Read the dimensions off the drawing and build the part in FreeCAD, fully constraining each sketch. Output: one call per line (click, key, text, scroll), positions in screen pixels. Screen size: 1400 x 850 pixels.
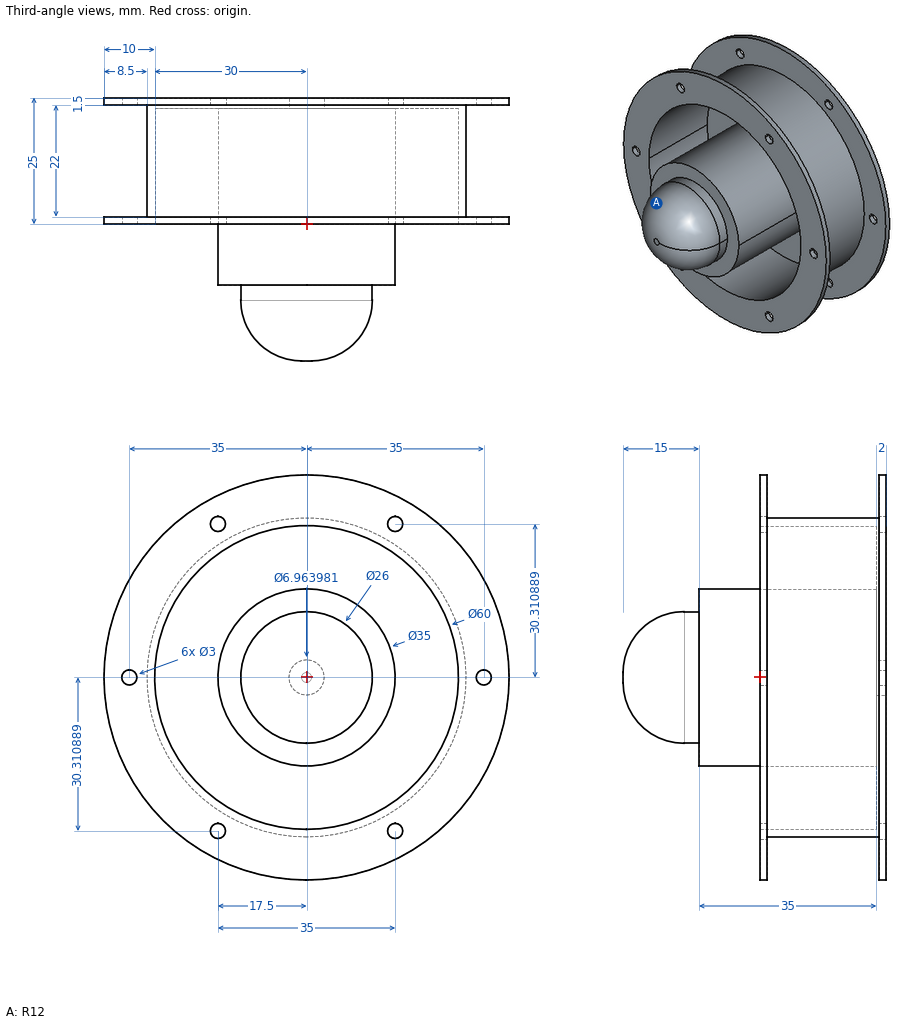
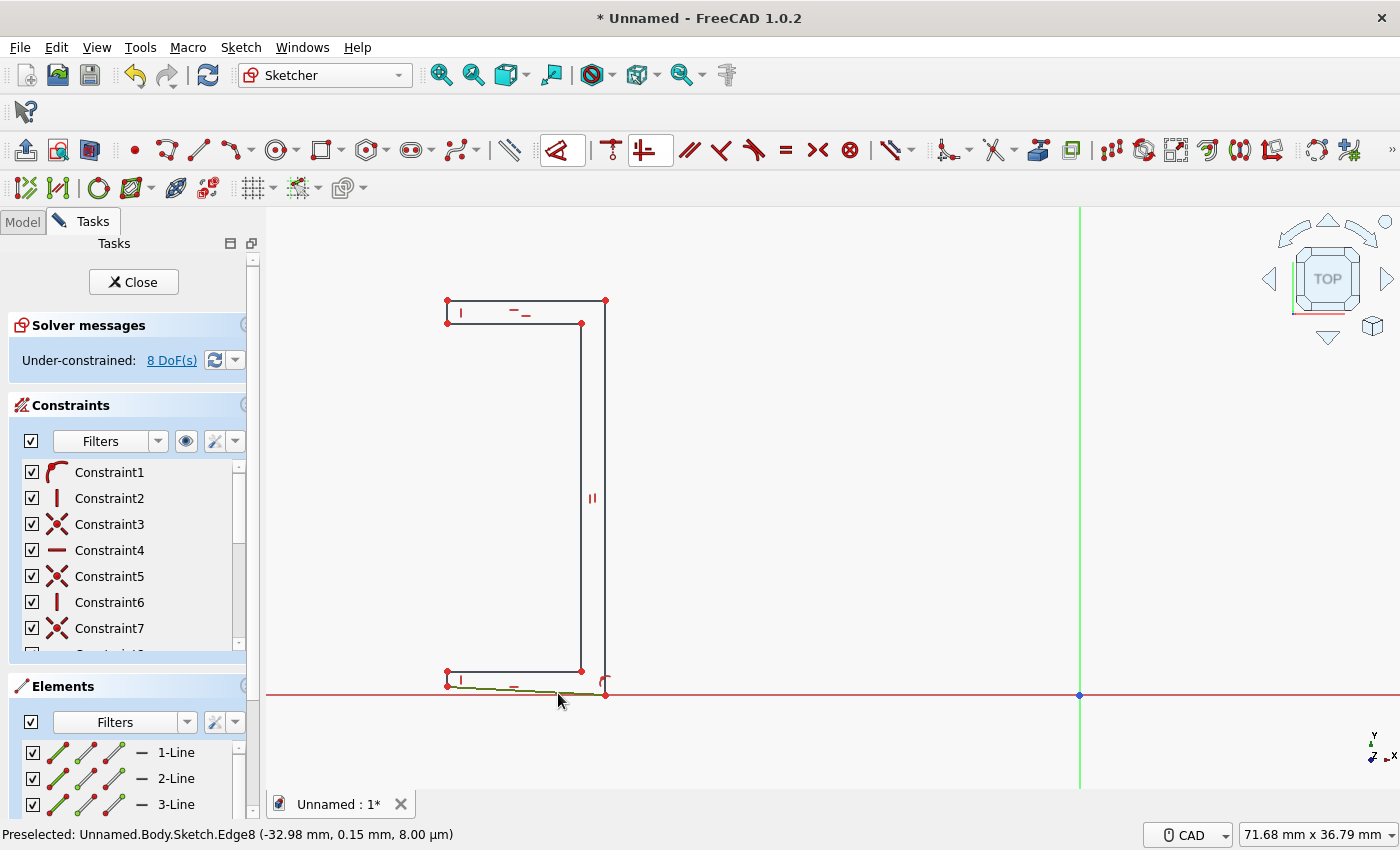
key(h)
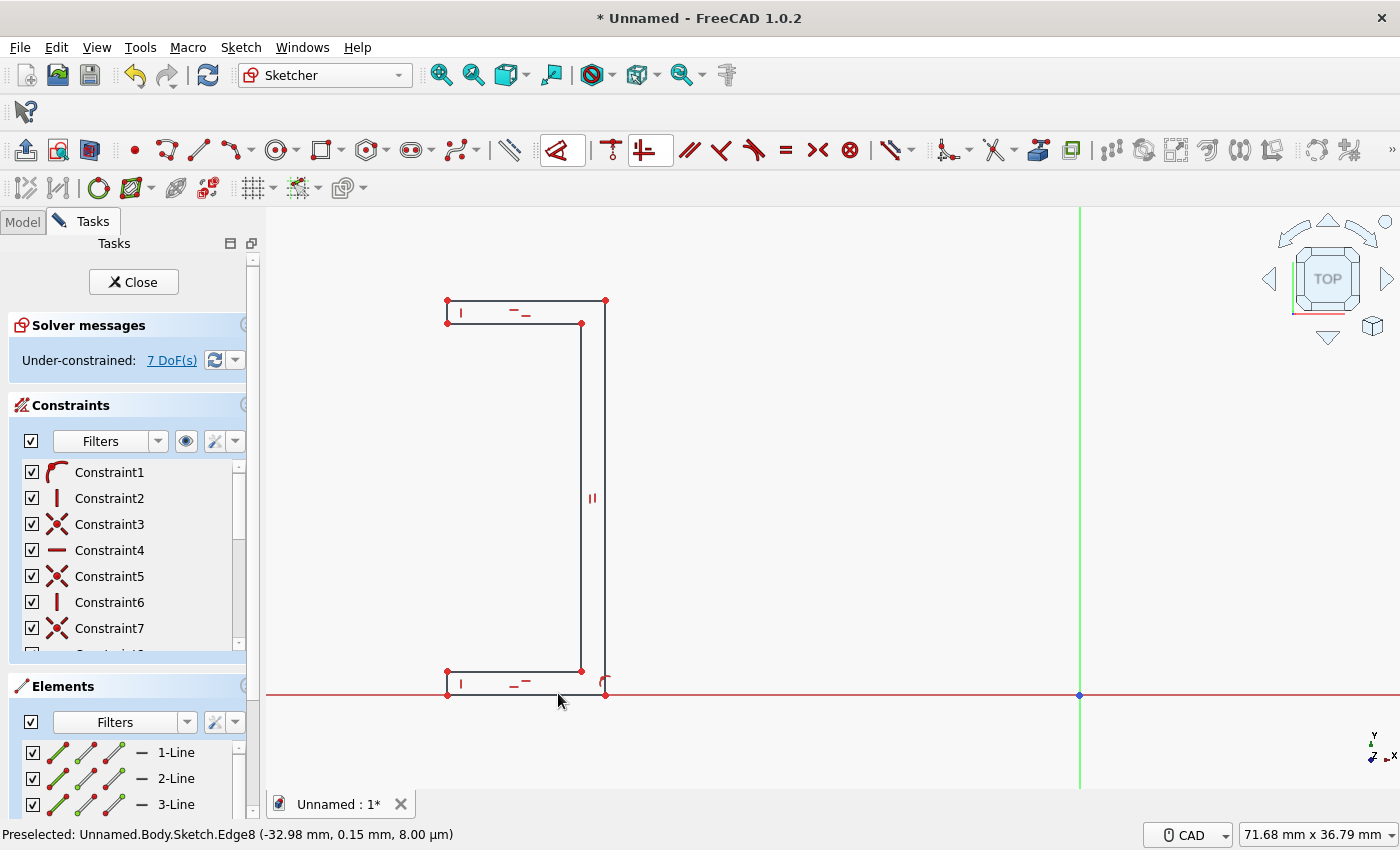
click(556, 150)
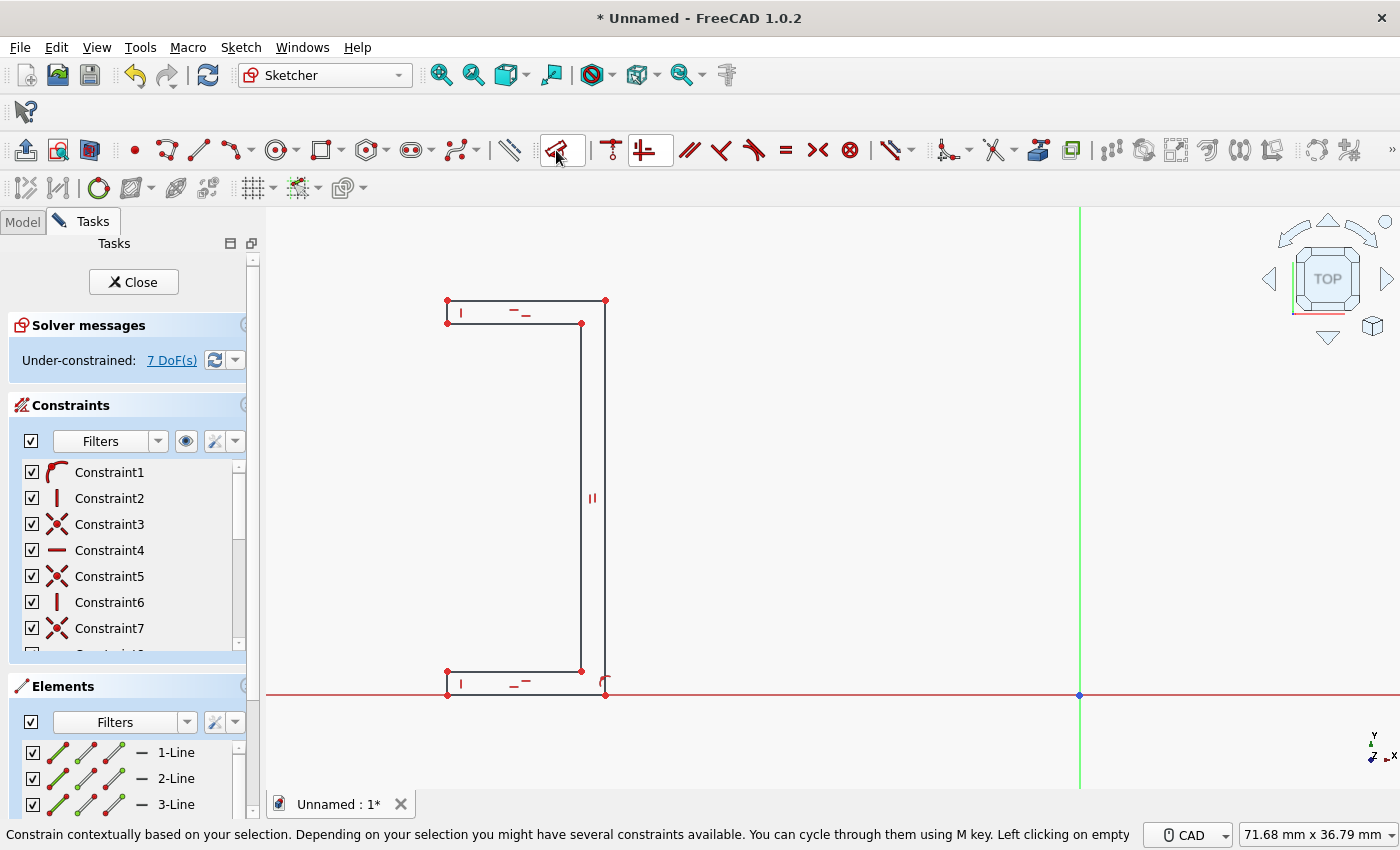
click(605, 577)
click(639, 498)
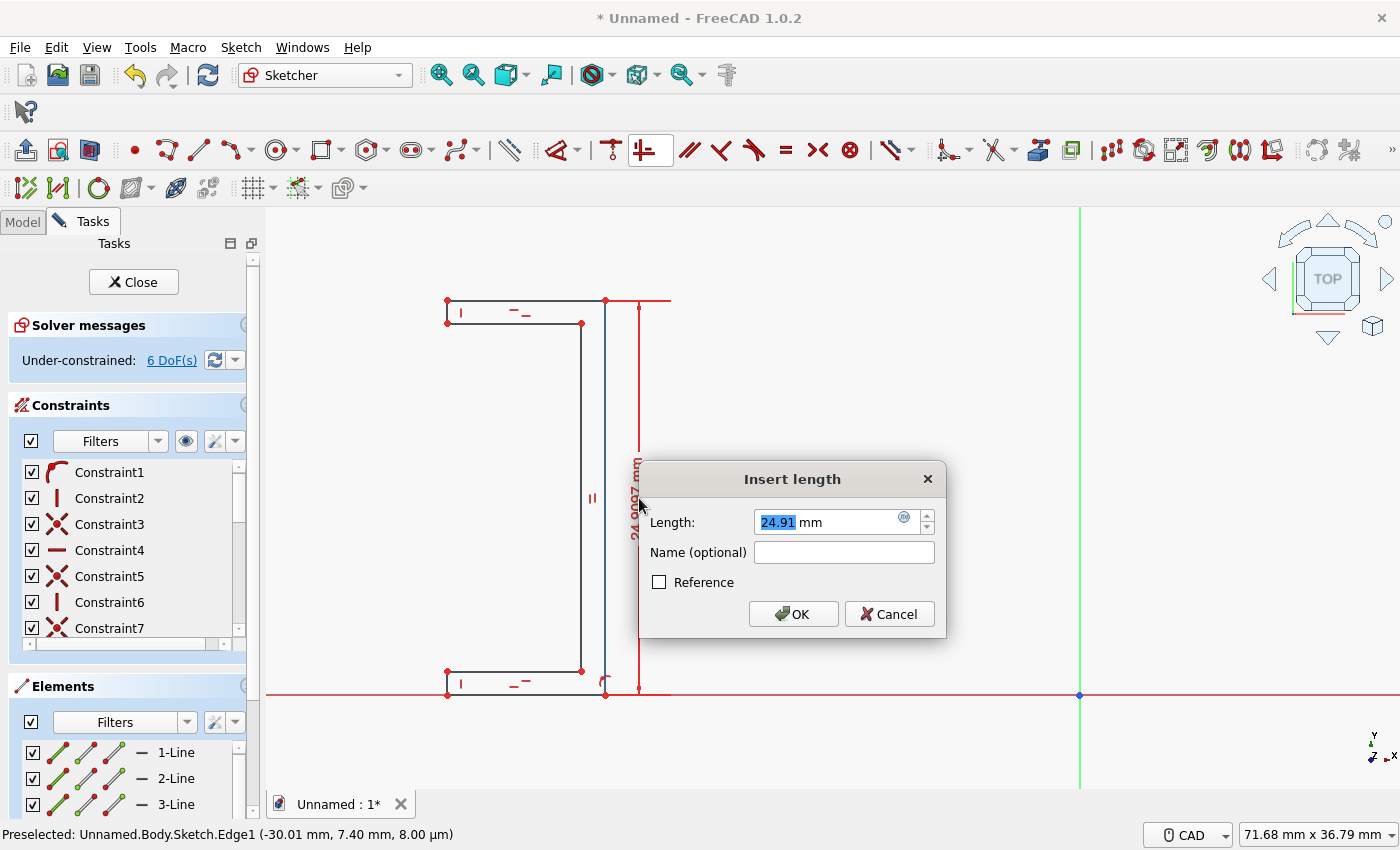
text(25)
key(Return)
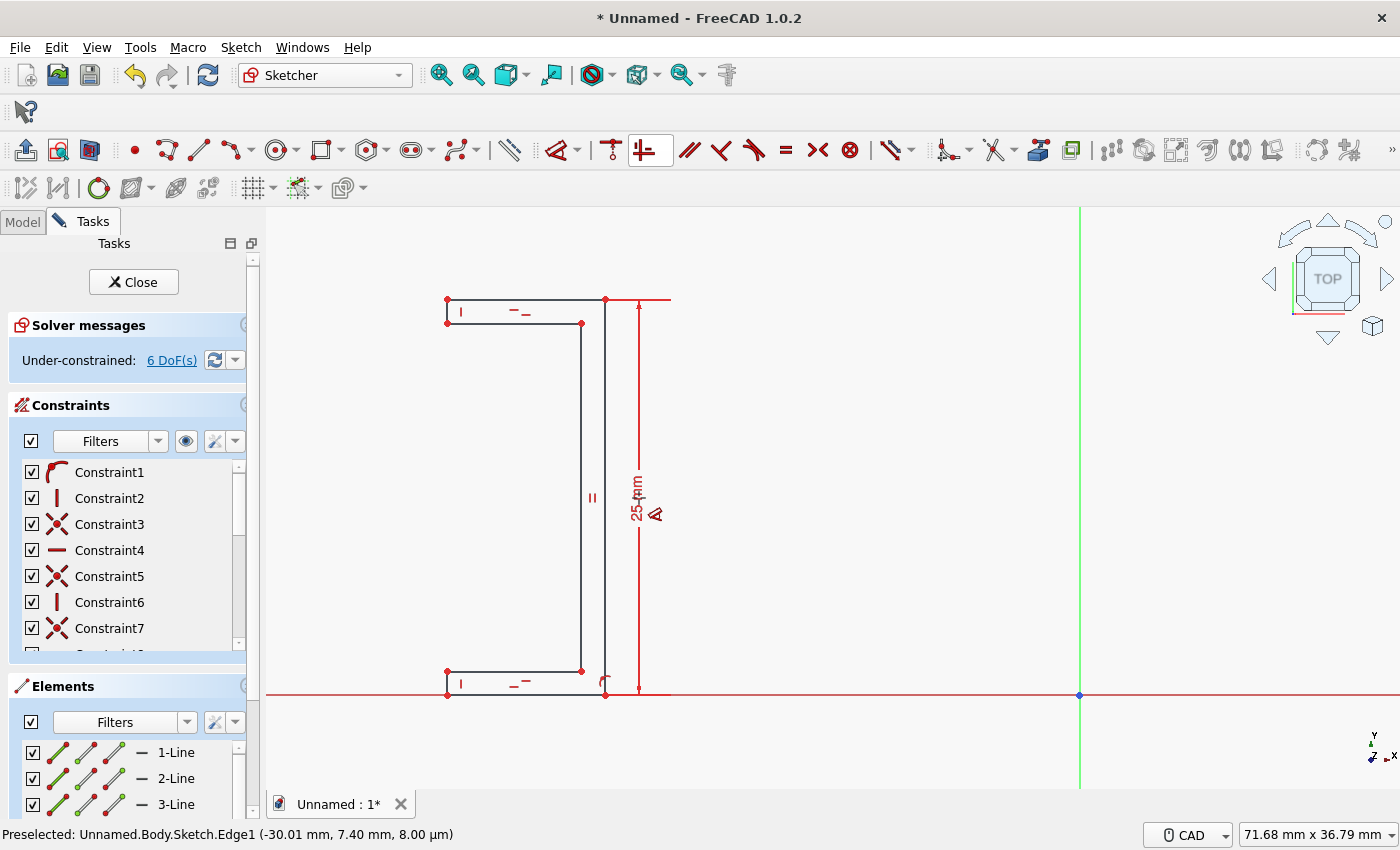
click(558, 300)
click(526, 266)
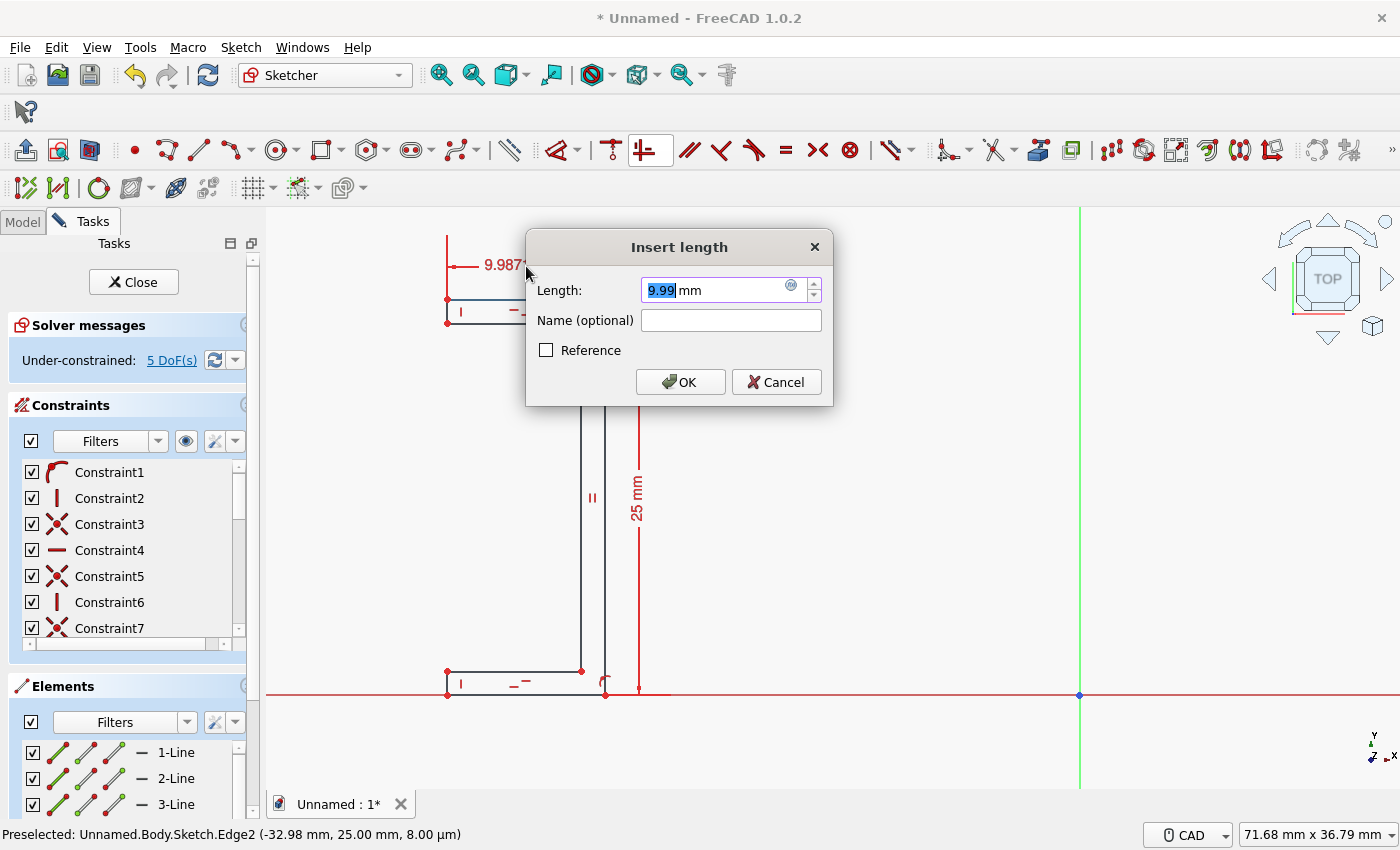
text(10)
key(Return)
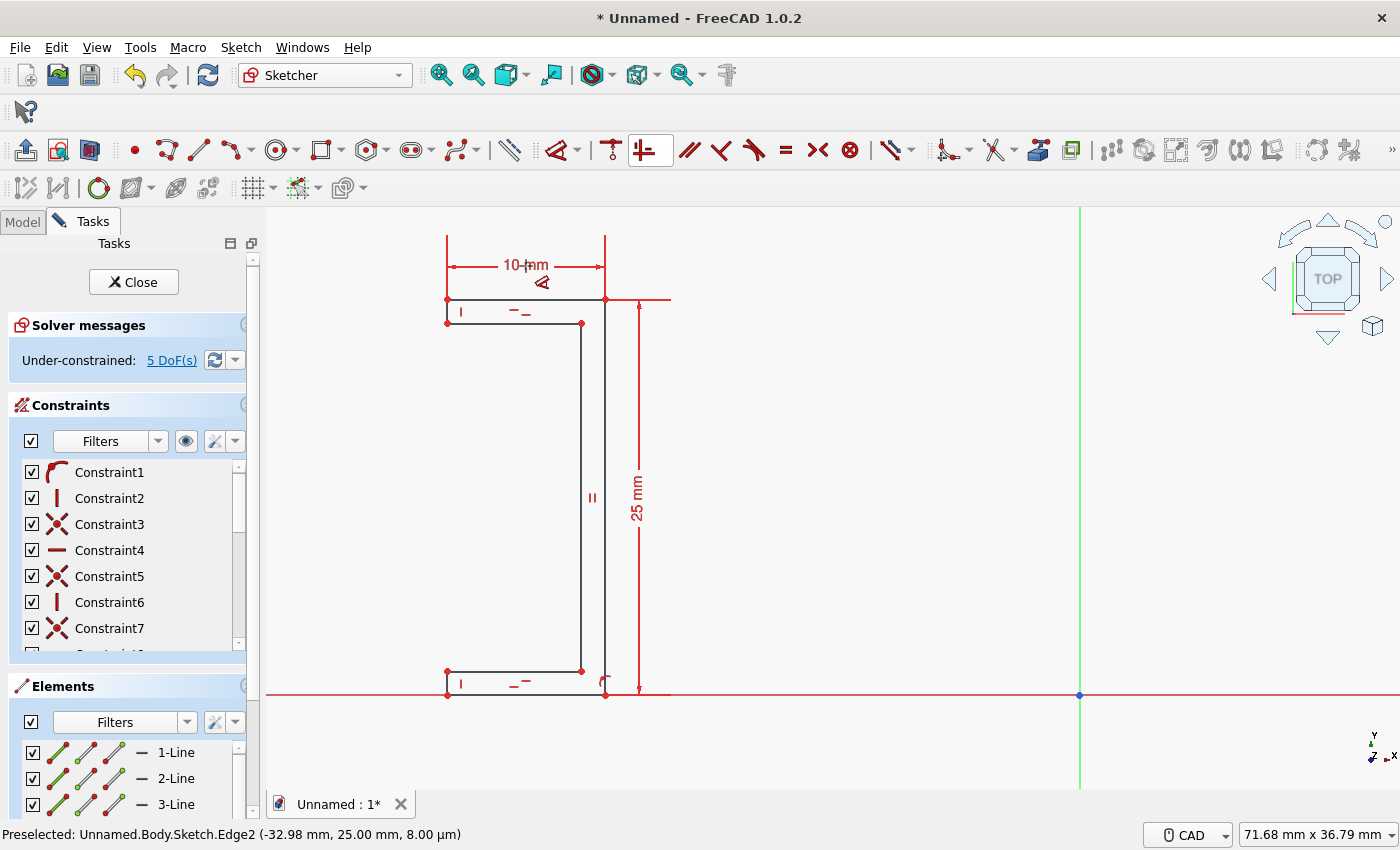
click(581, 428)
click(547, 498)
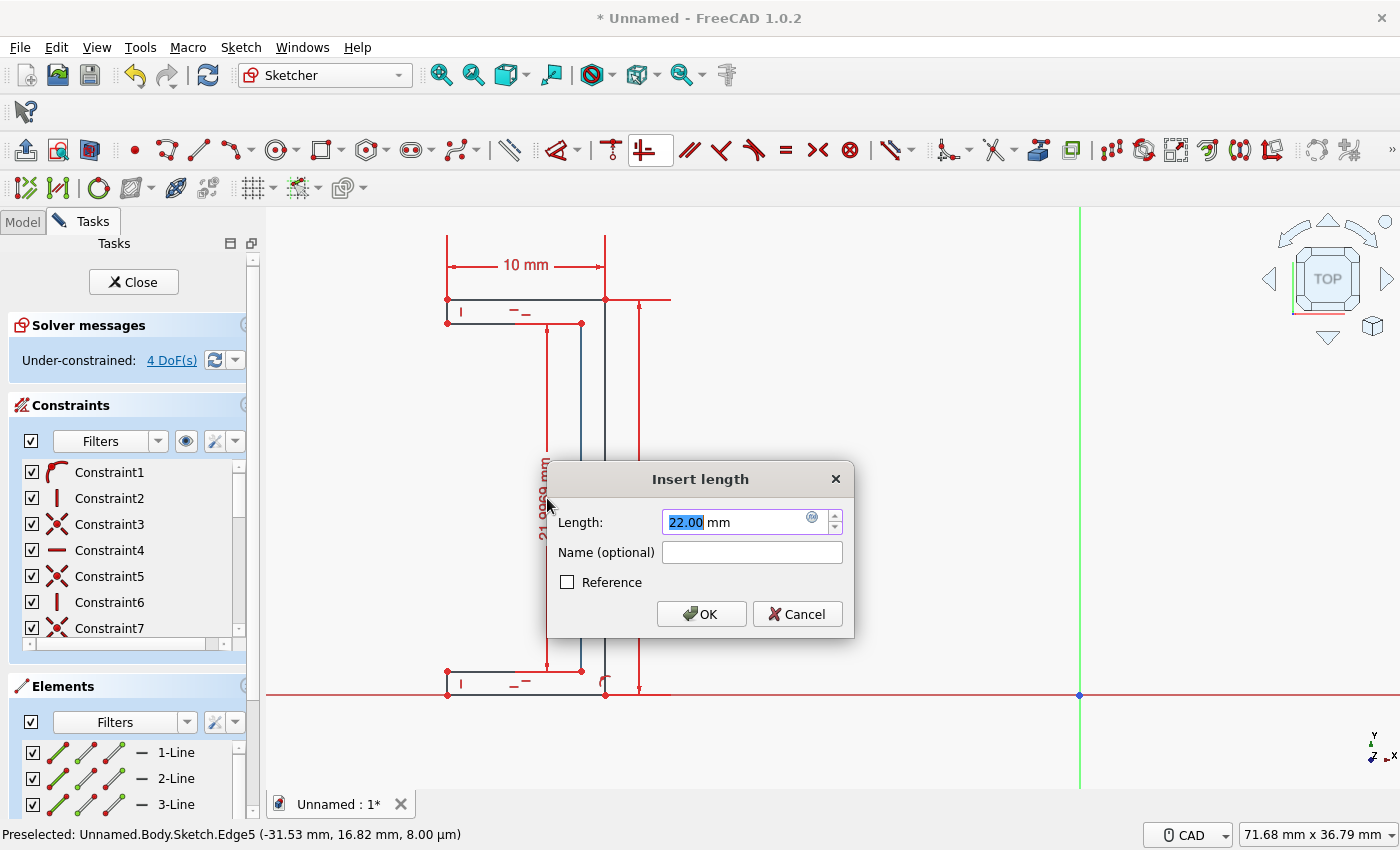
text(22)
key(Return)